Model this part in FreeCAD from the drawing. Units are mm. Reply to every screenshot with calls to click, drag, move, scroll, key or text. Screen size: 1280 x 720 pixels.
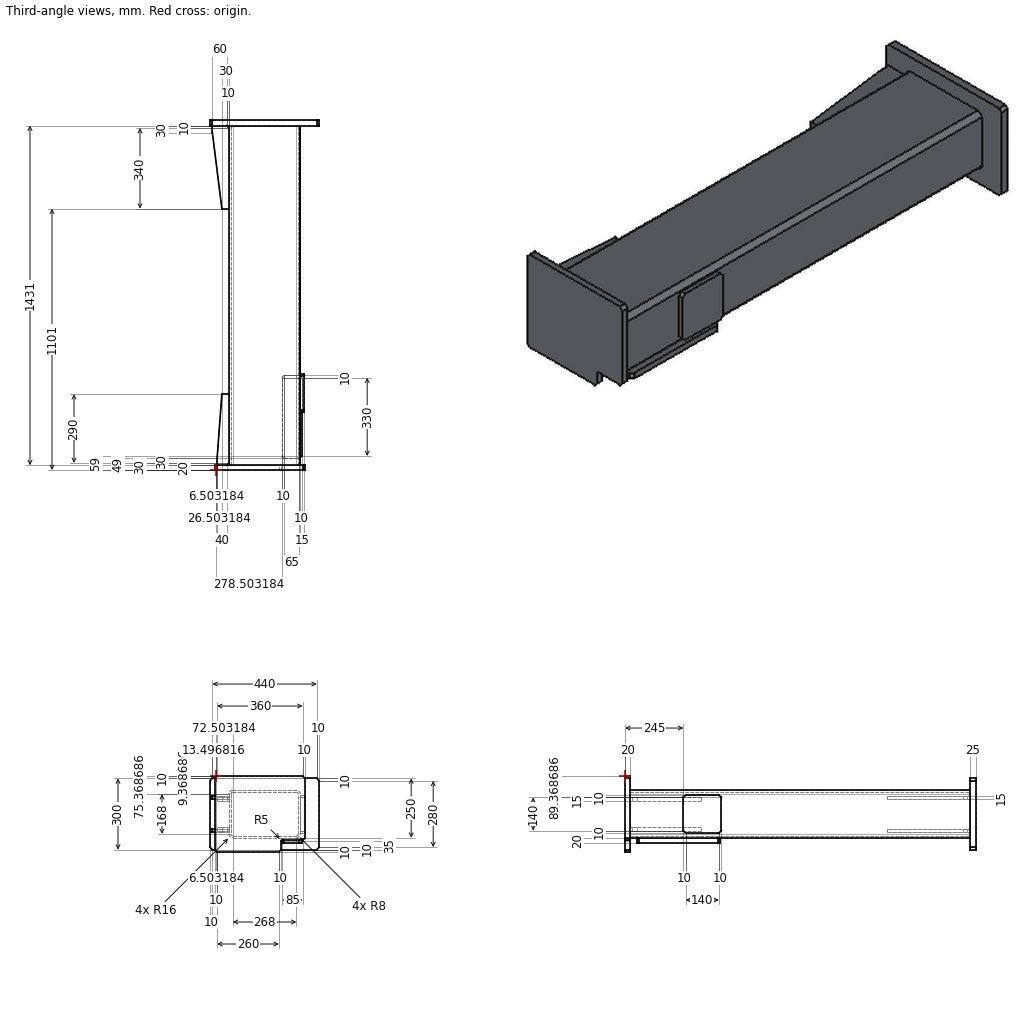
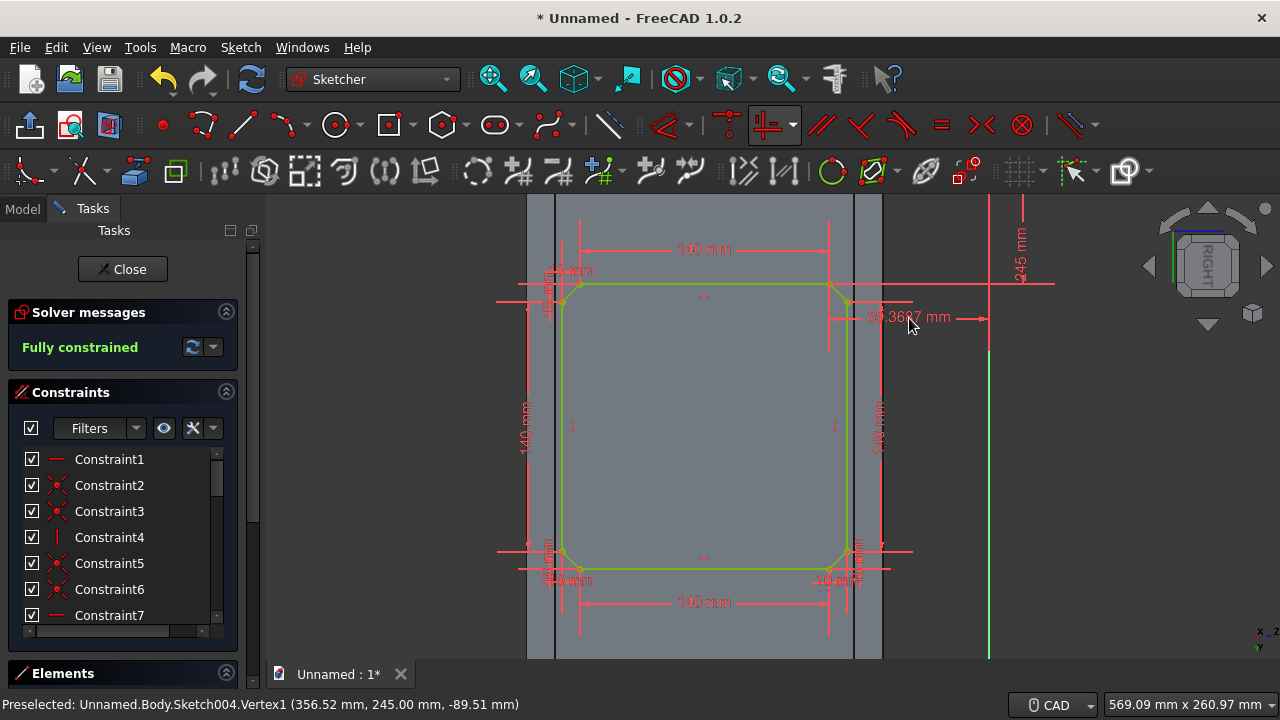
click(123, 269)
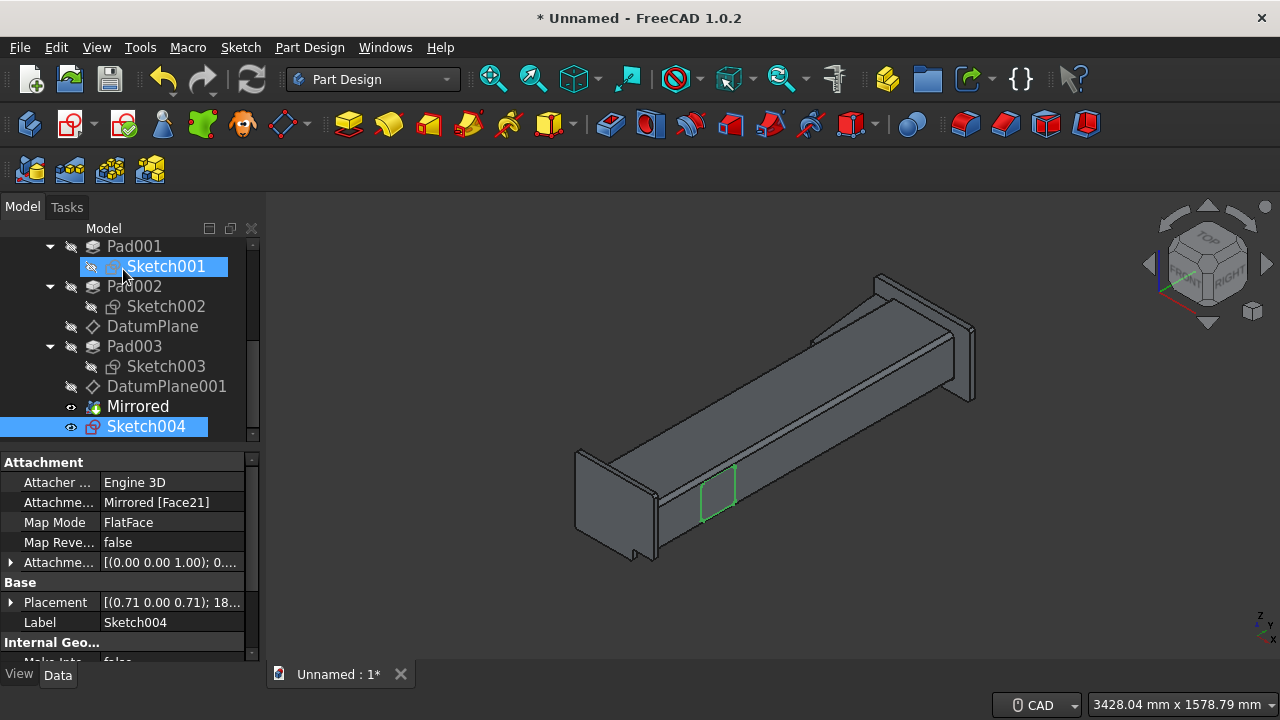
click(350, 124)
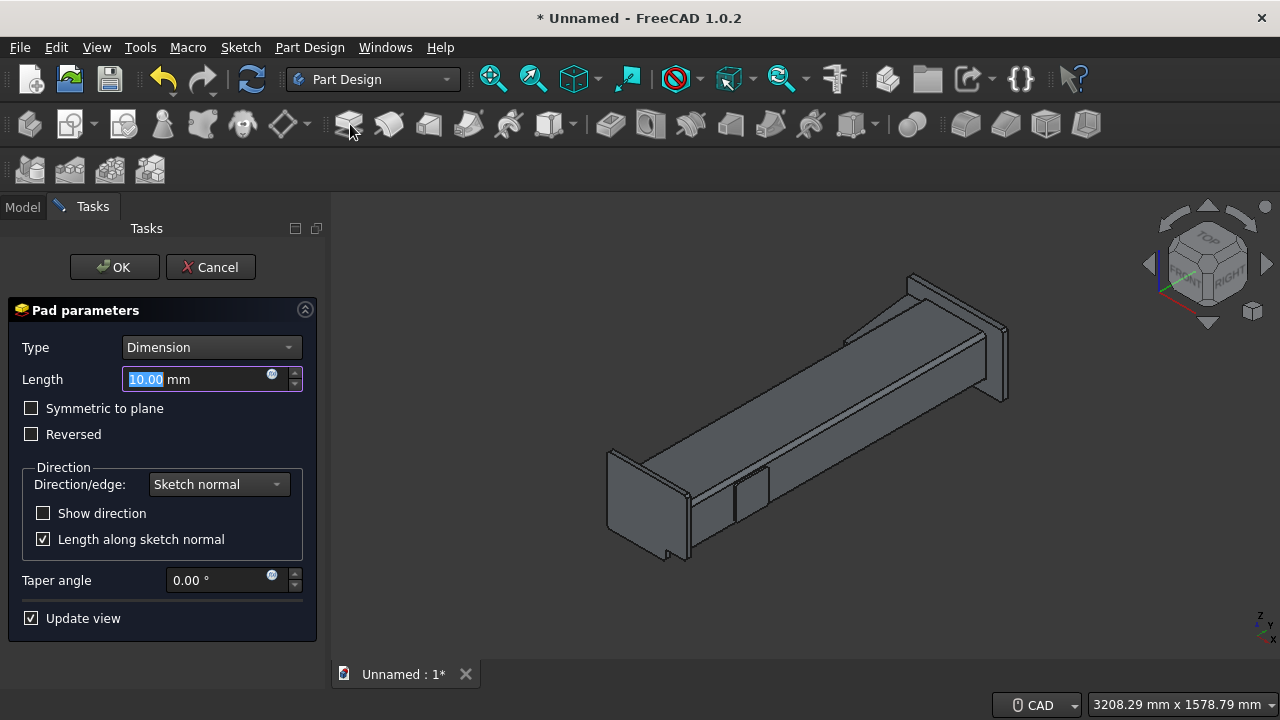
text(15)
key(Tab)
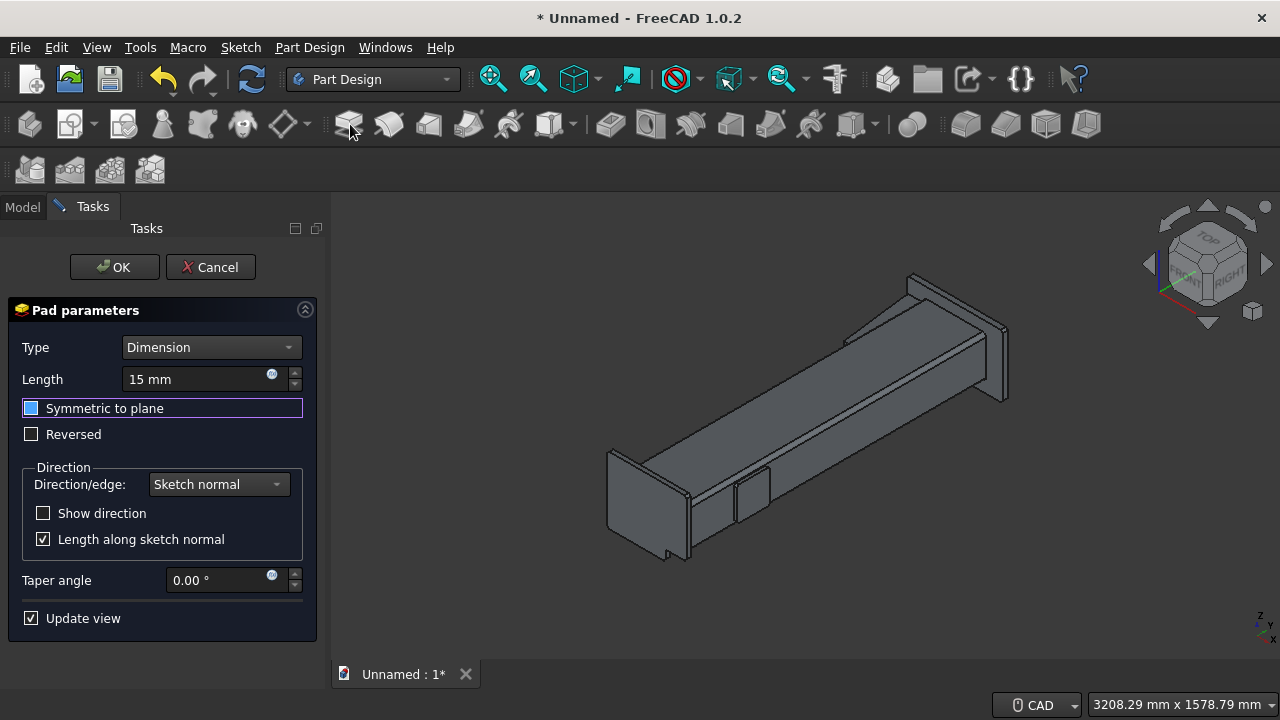
click(115, 267)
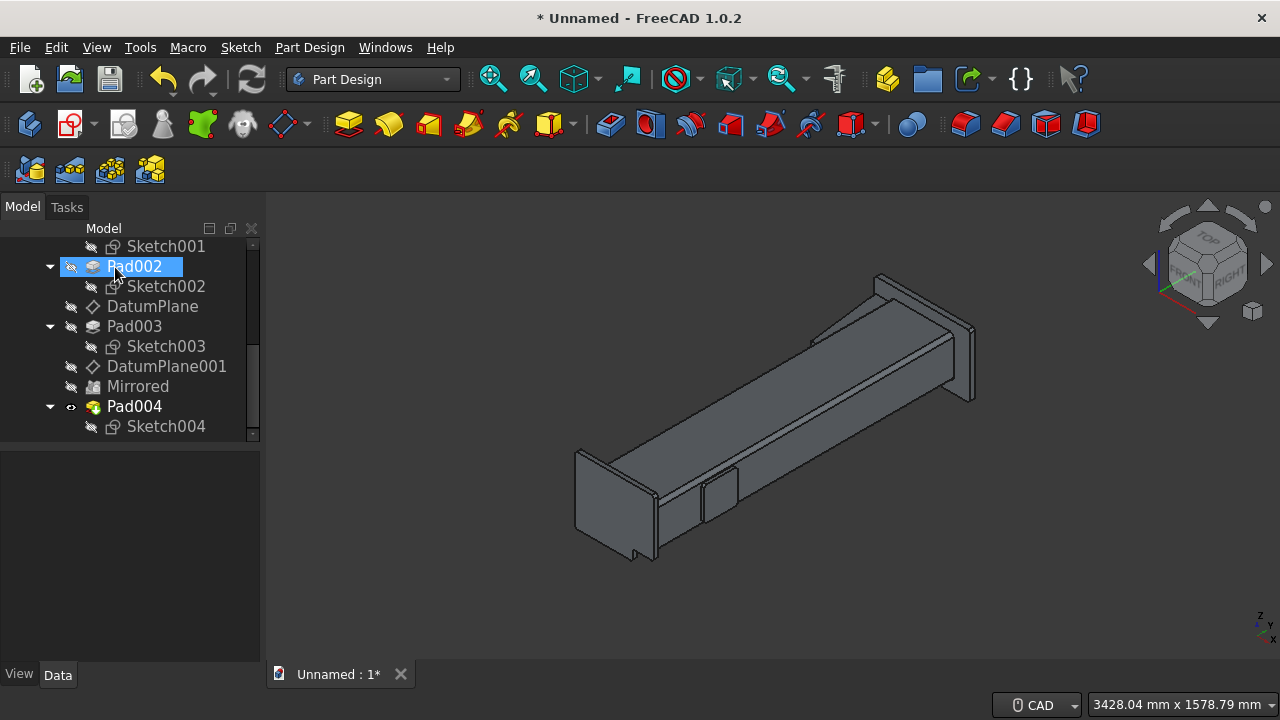
scroll(160, 342, down, 3)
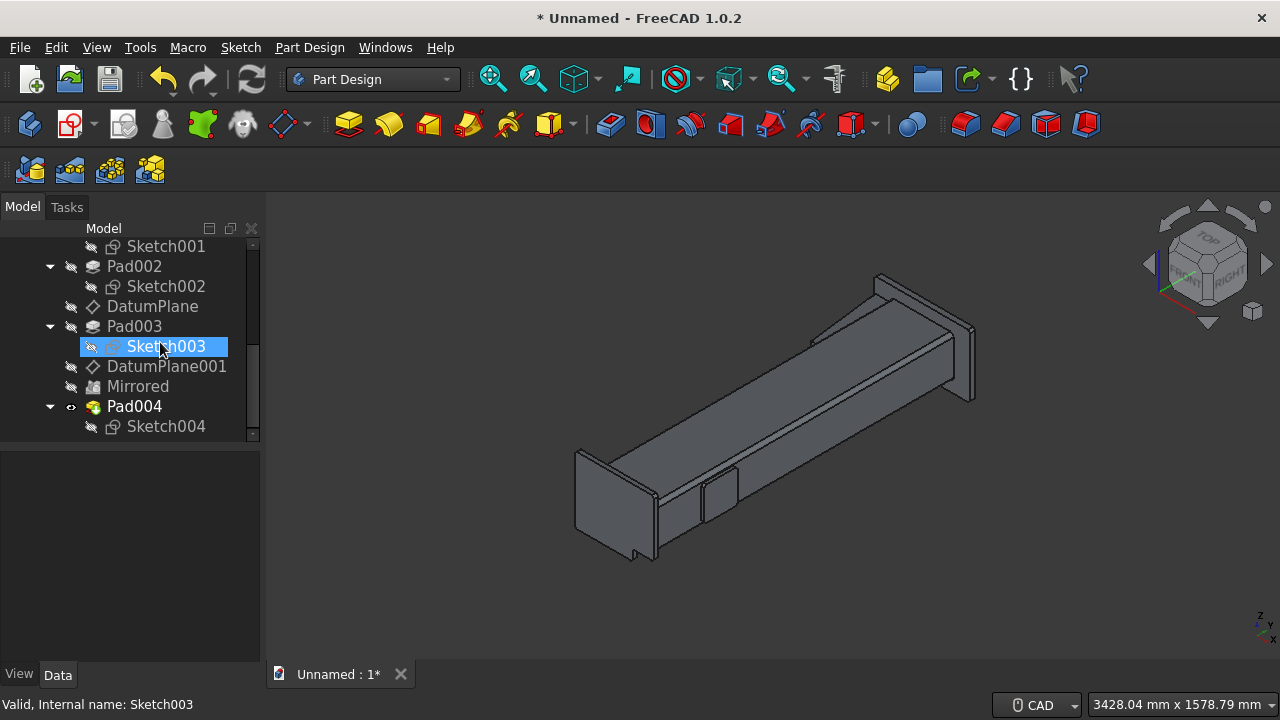
scroll(160, 342, up, 15)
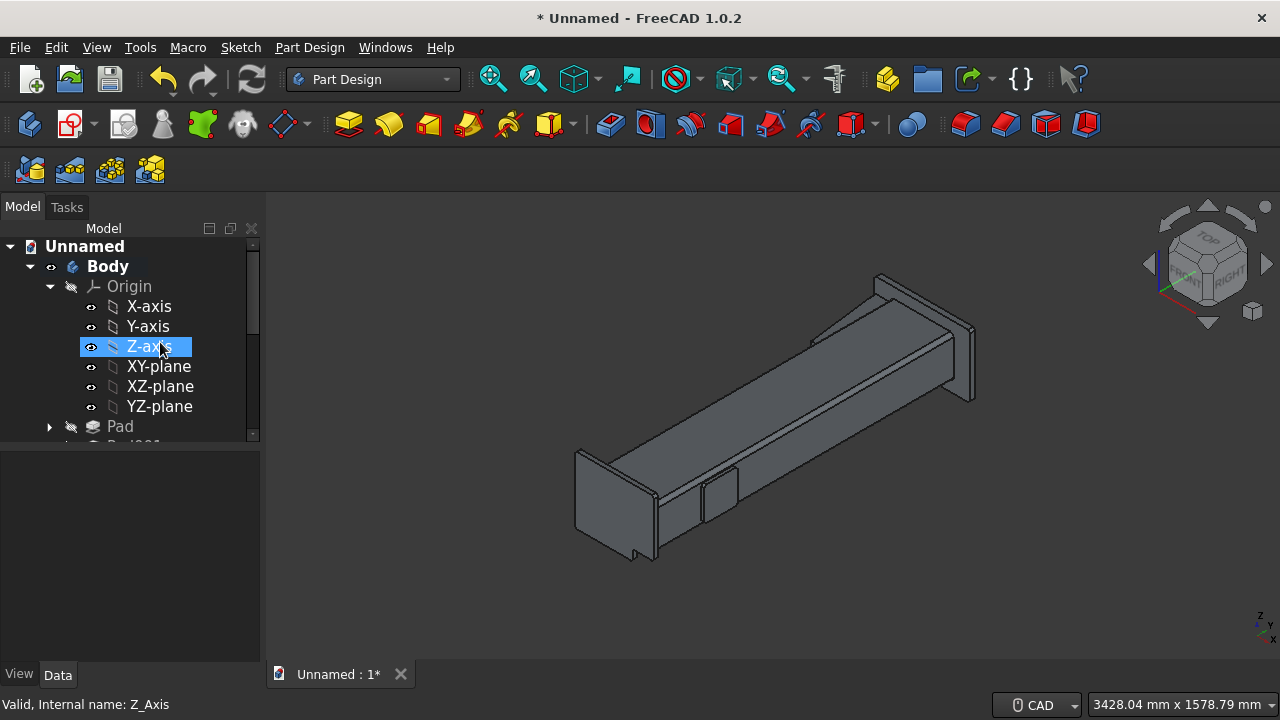
click(136, 367)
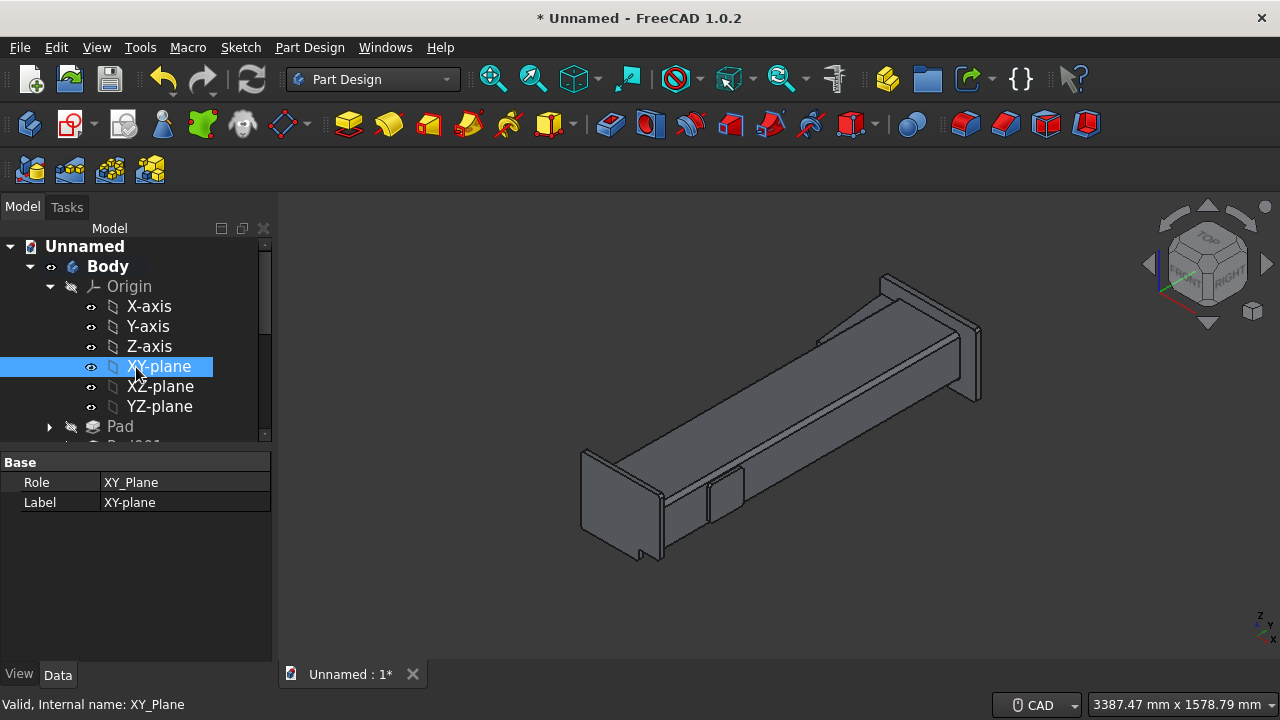
click(284, 124)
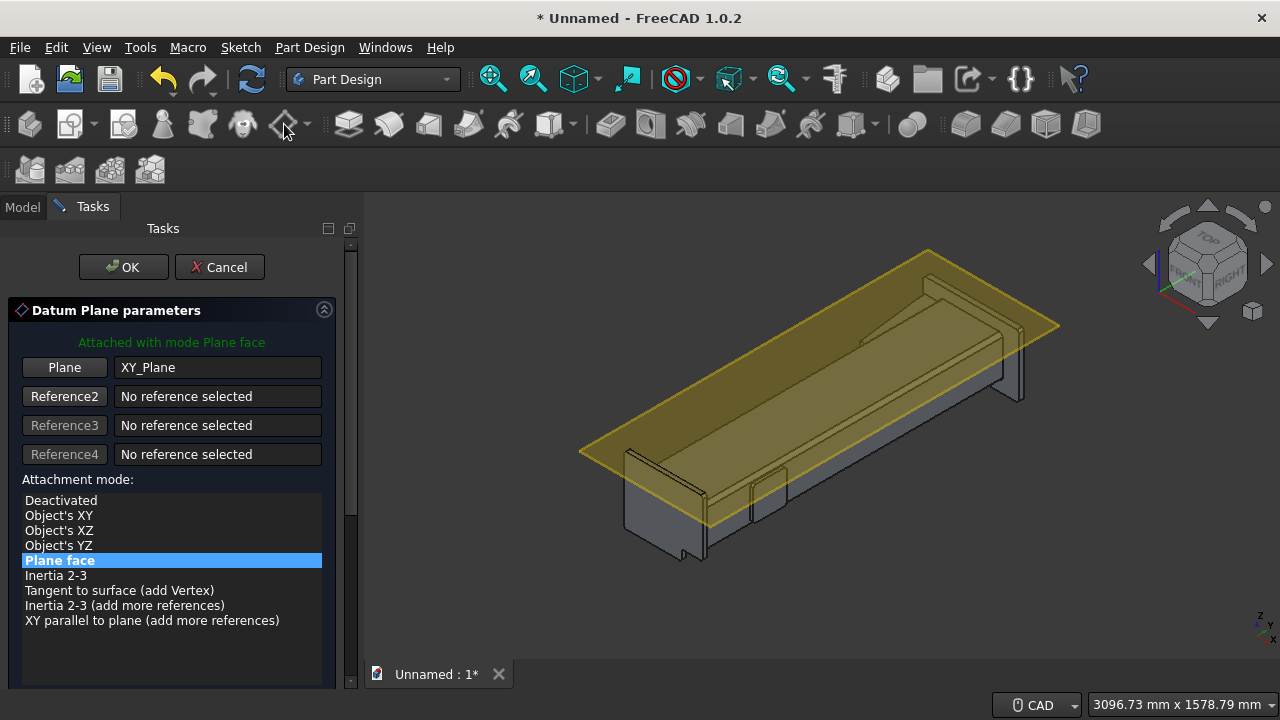
scroll(351, 463, down, 3)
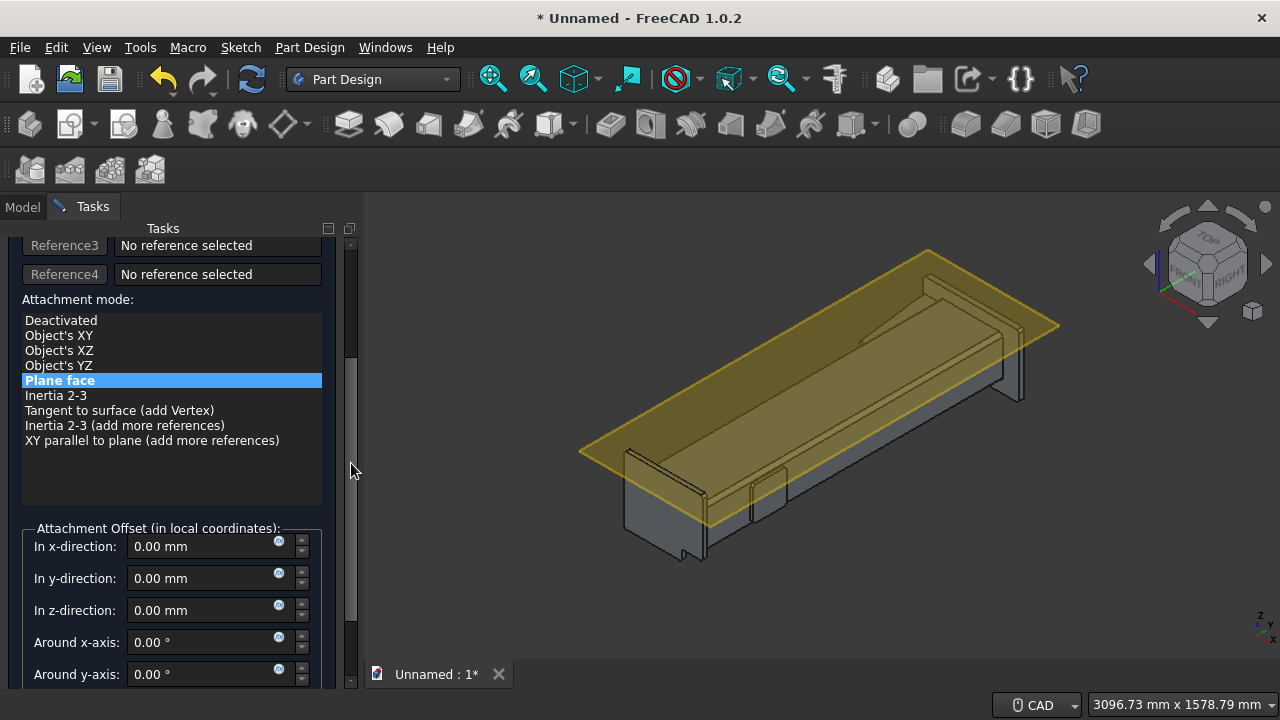
triple_click(210, 610)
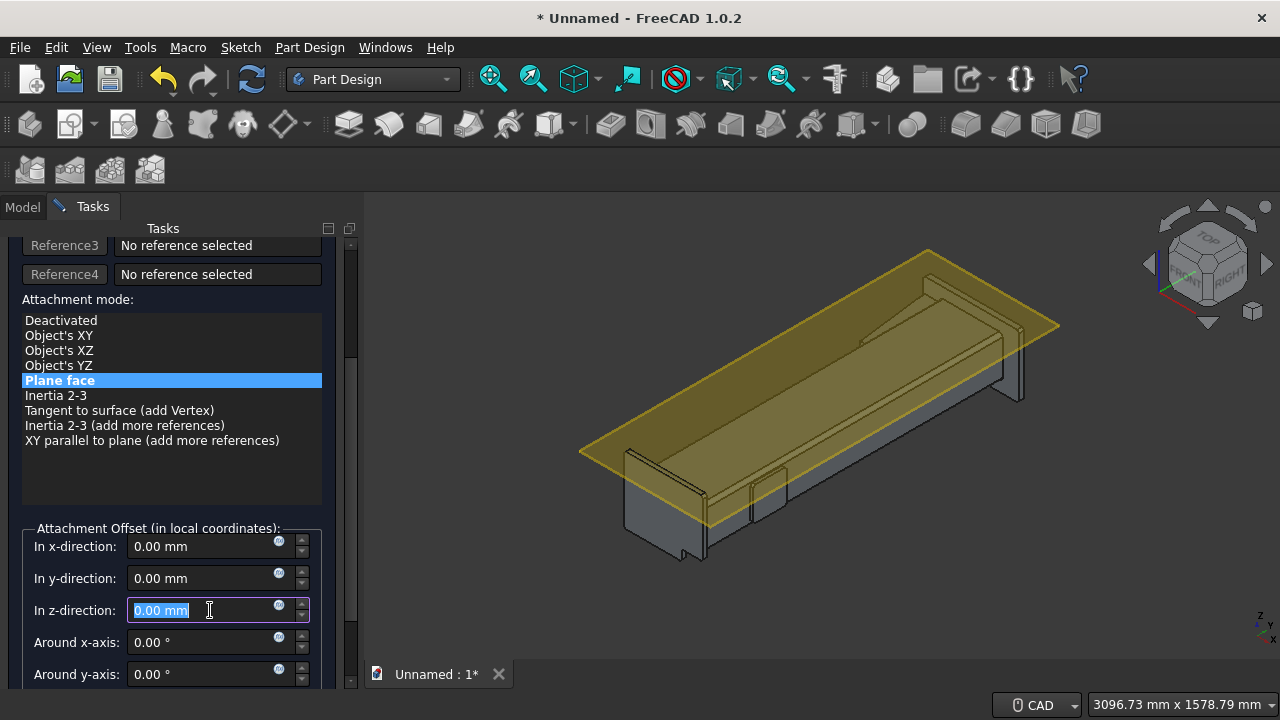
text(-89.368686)
key(Tab)